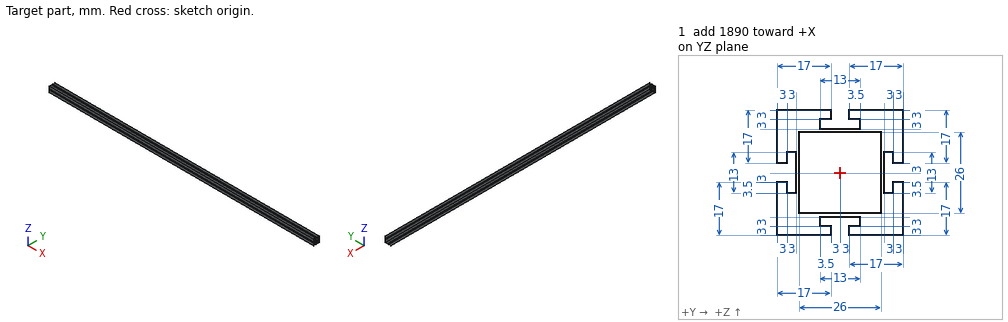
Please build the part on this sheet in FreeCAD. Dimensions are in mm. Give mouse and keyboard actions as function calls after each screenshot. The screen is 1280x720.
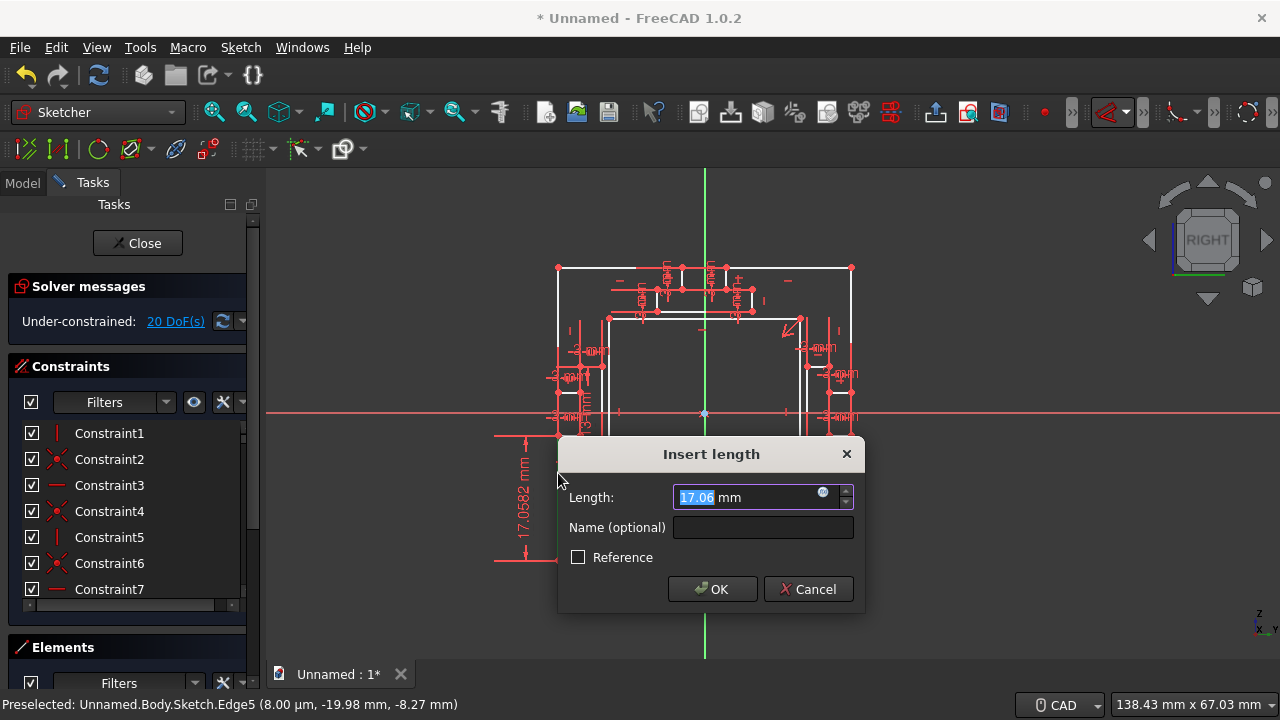
text(17)
key(Return)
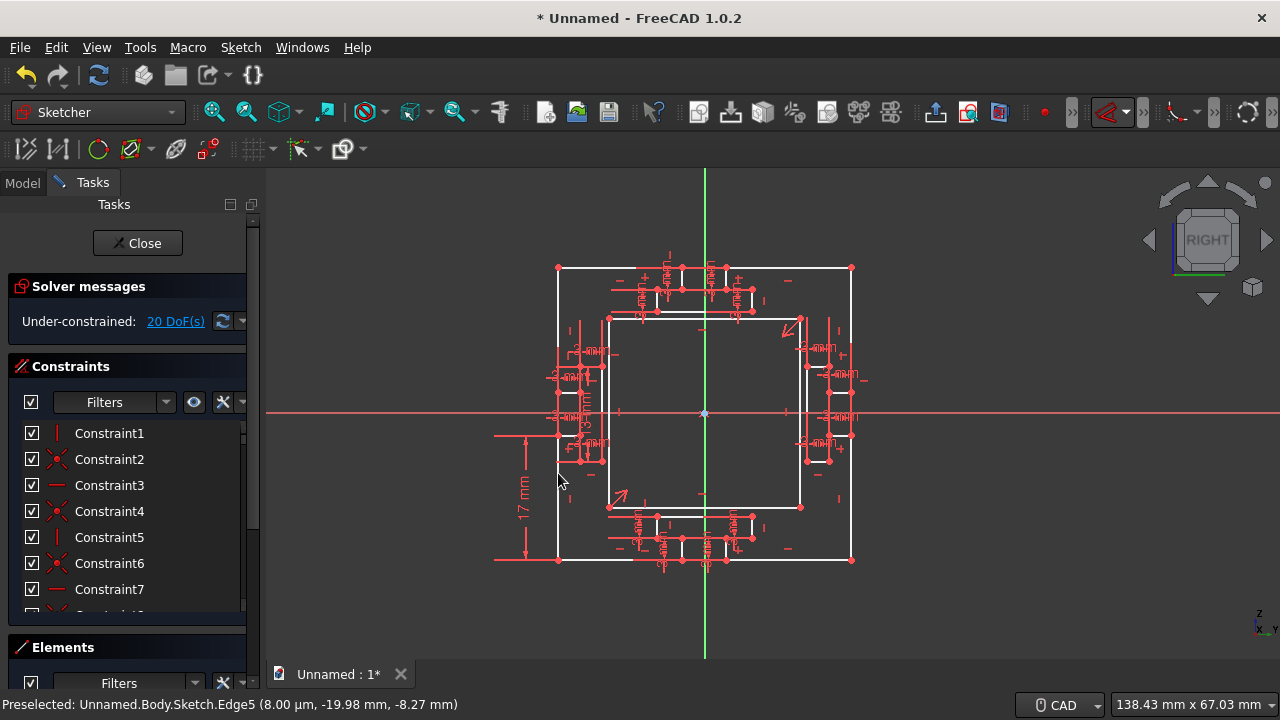
click(596, 560)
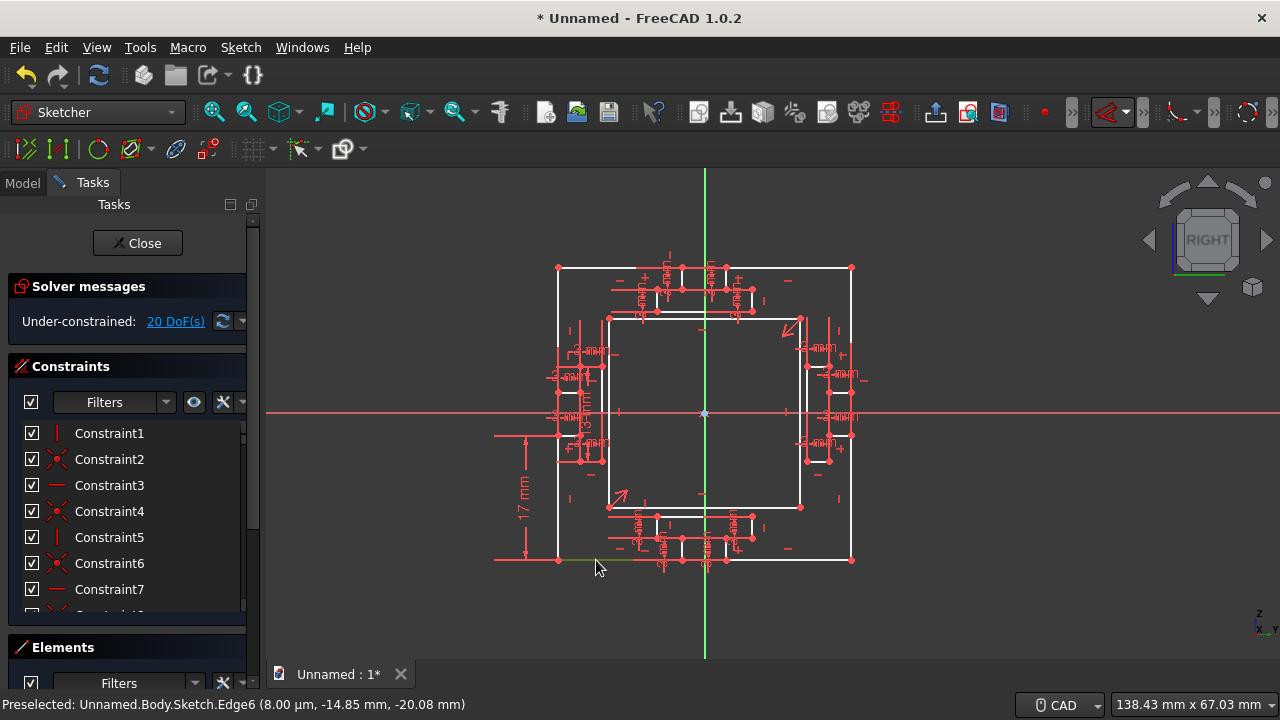
click(1128, 112)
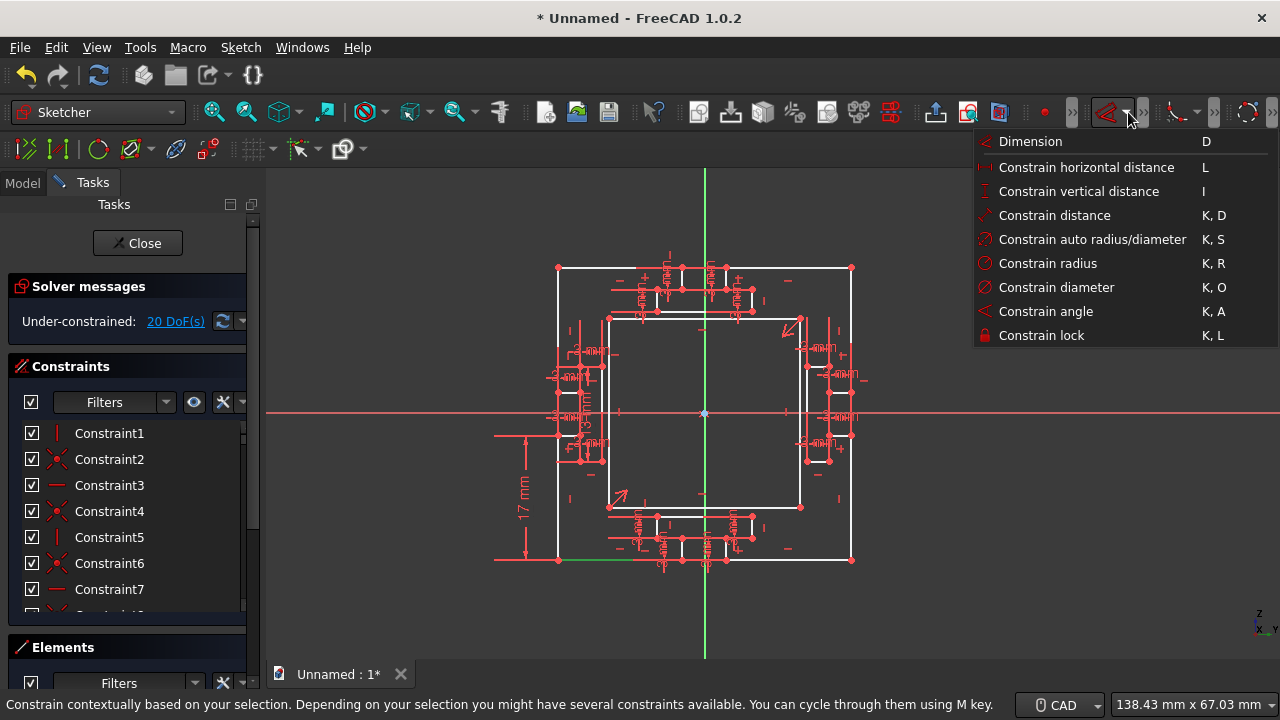
click(1126, 167)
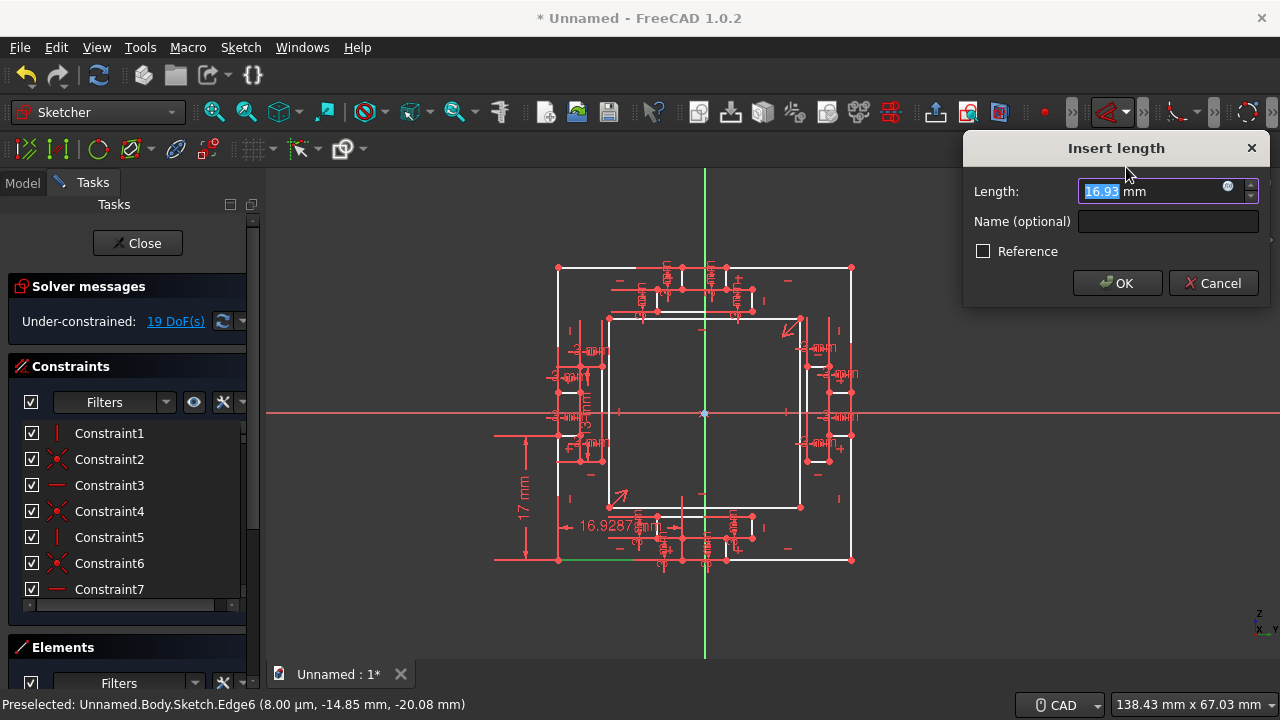
text(17)
key(Return)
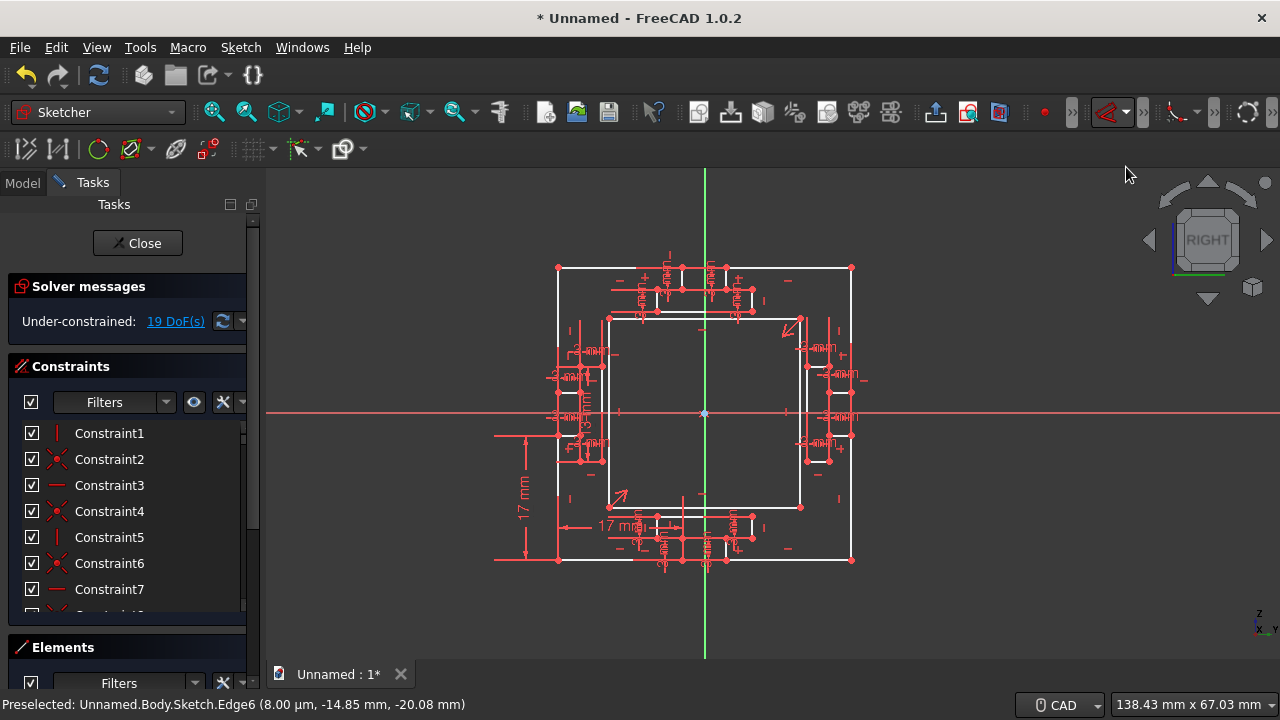
scroll(686, 517, up, 3)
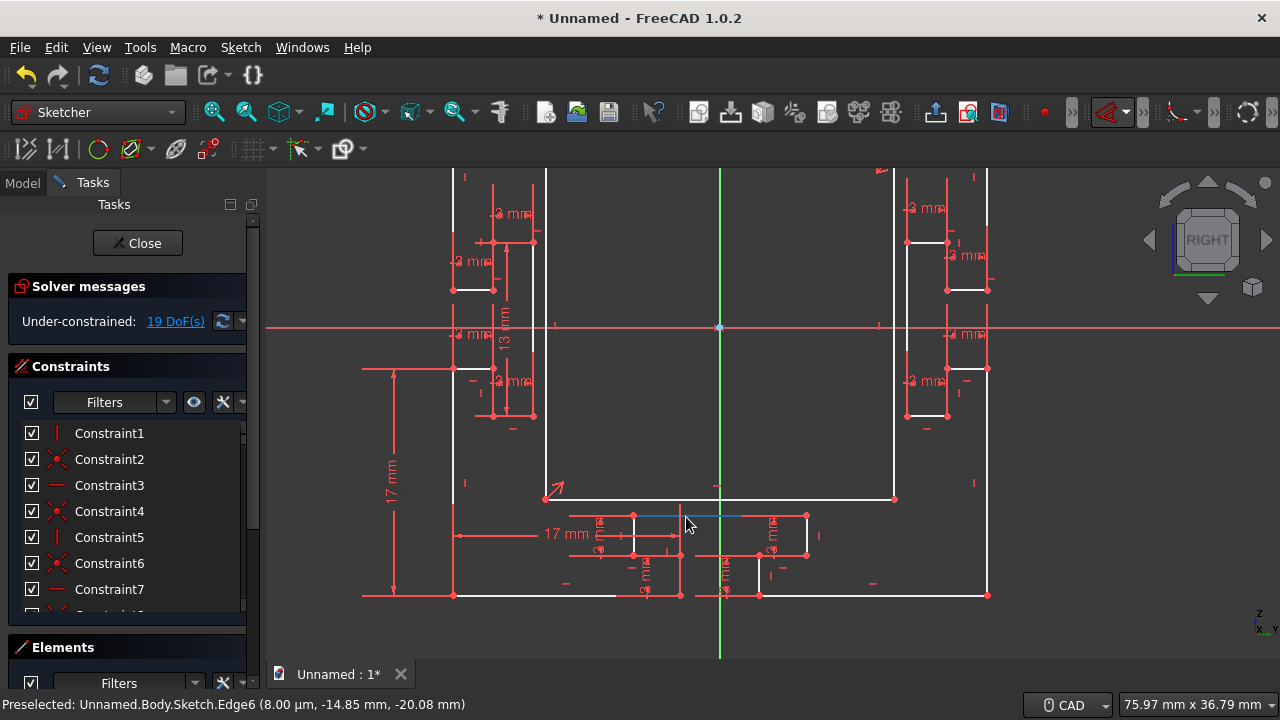
click(686, 516)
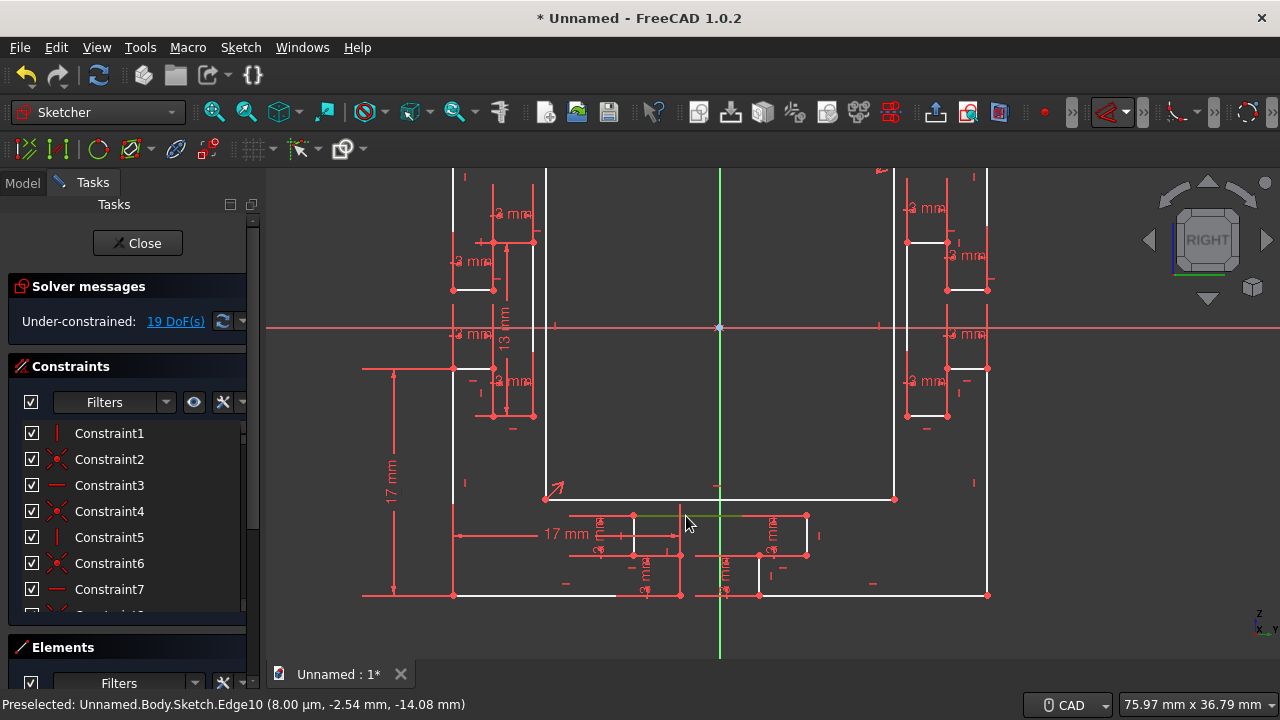
key(l)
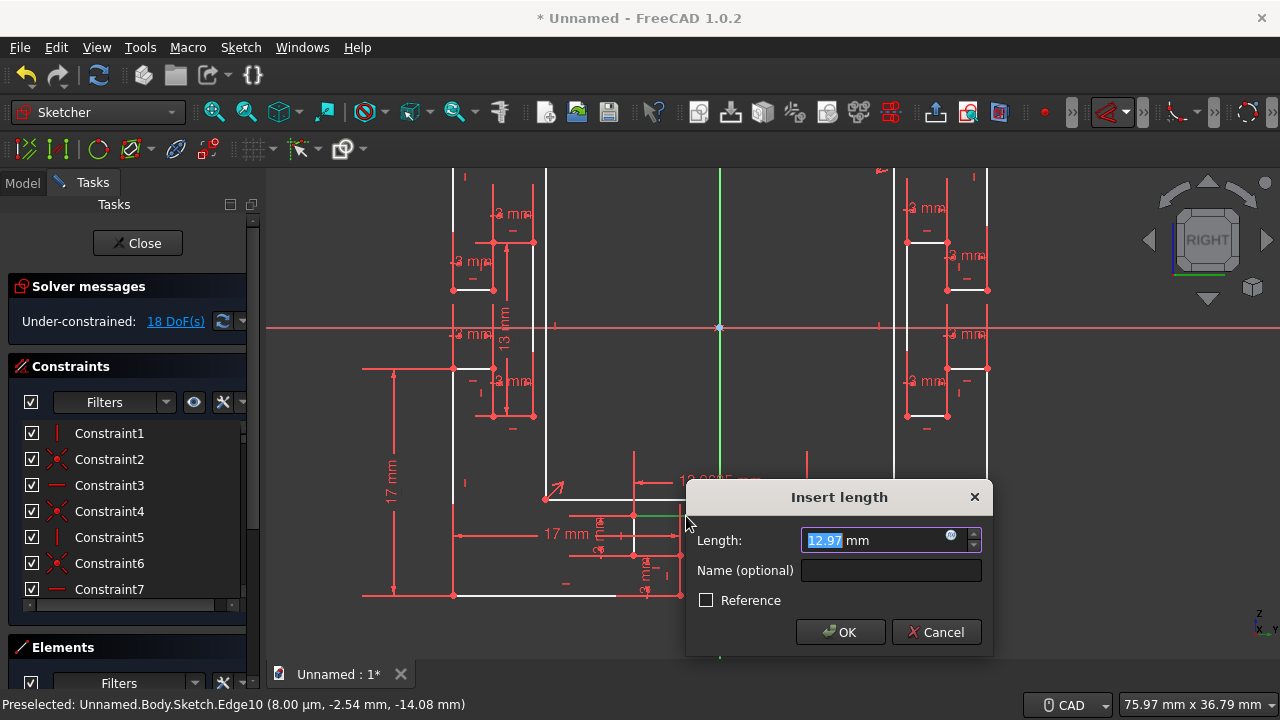
text(13)
key(Return)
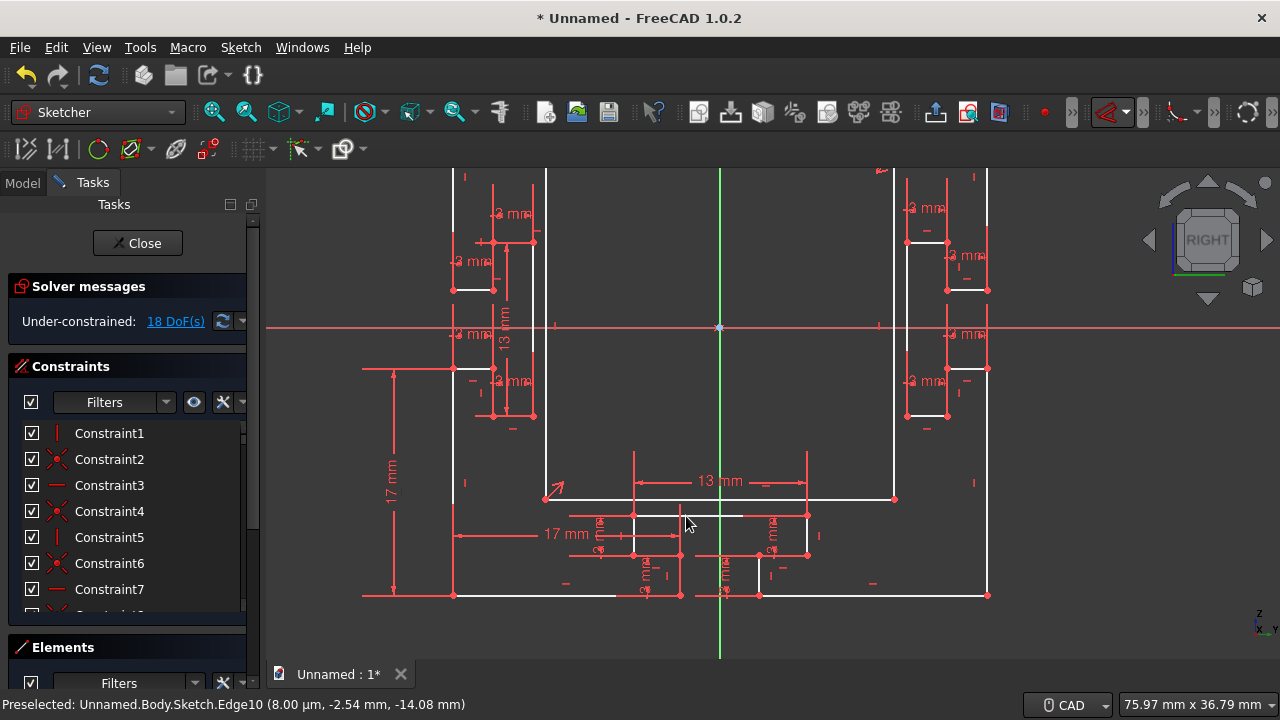
click(828, 596)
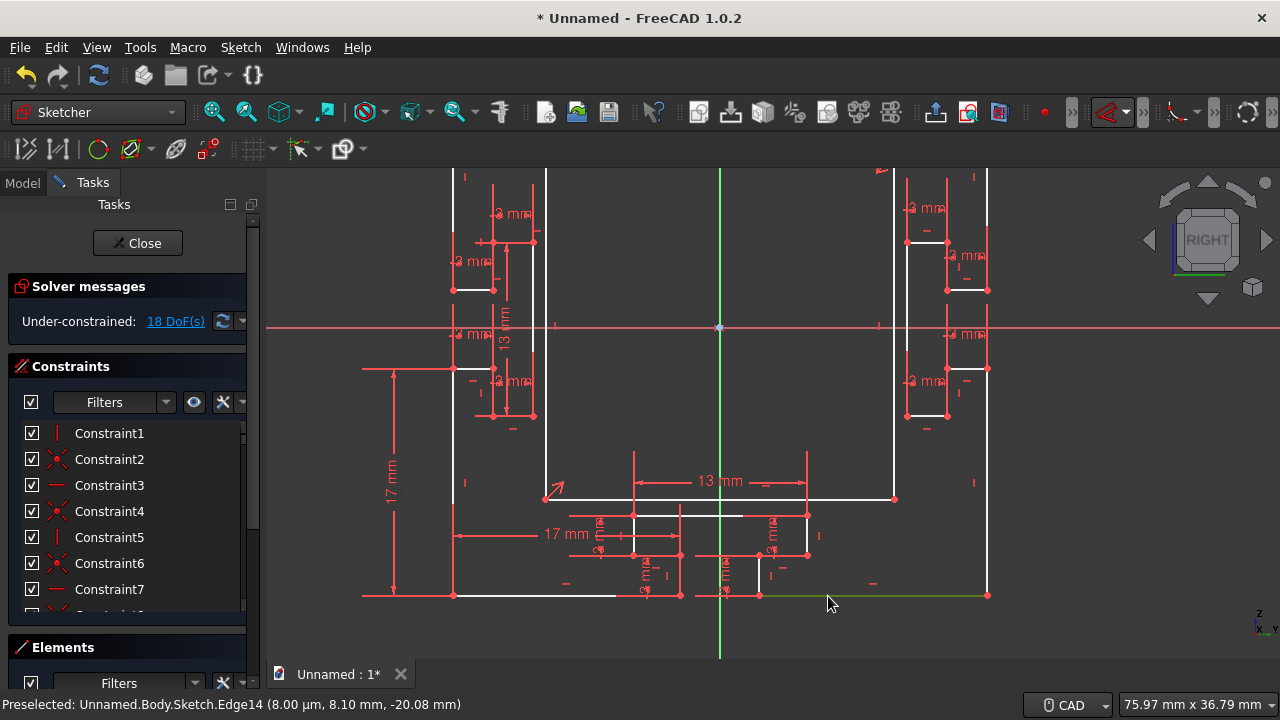
key(l)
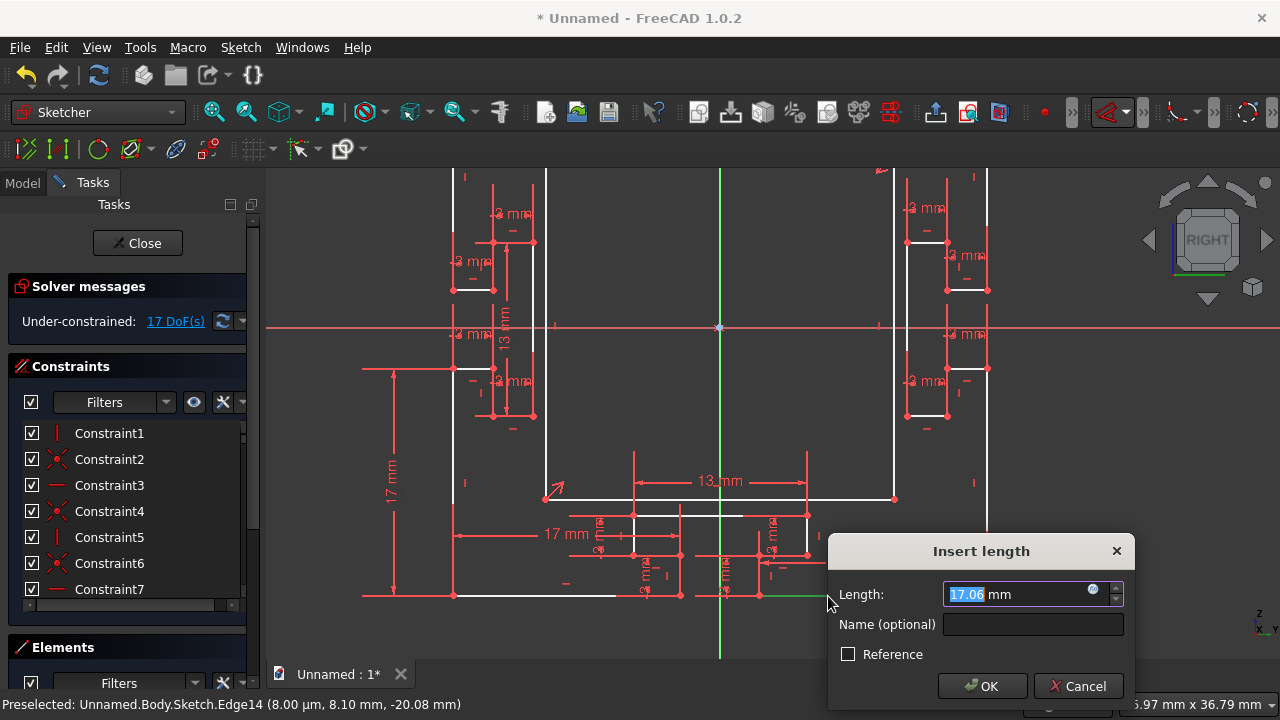
text(17)
key(Return)